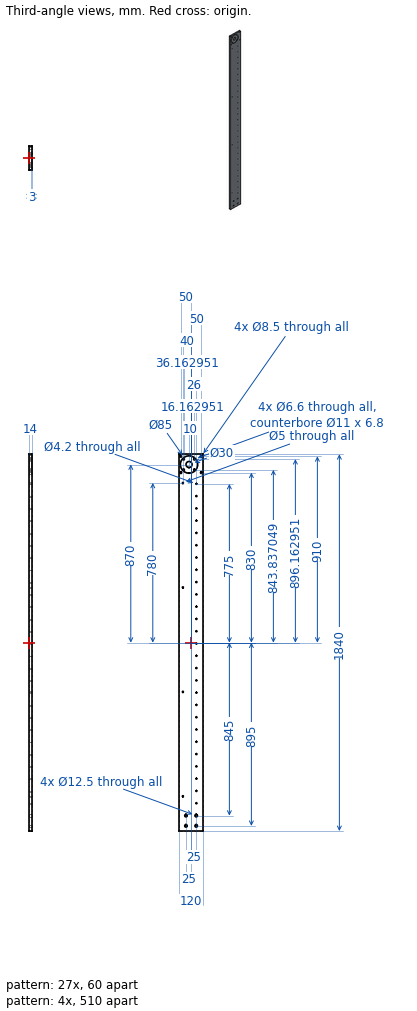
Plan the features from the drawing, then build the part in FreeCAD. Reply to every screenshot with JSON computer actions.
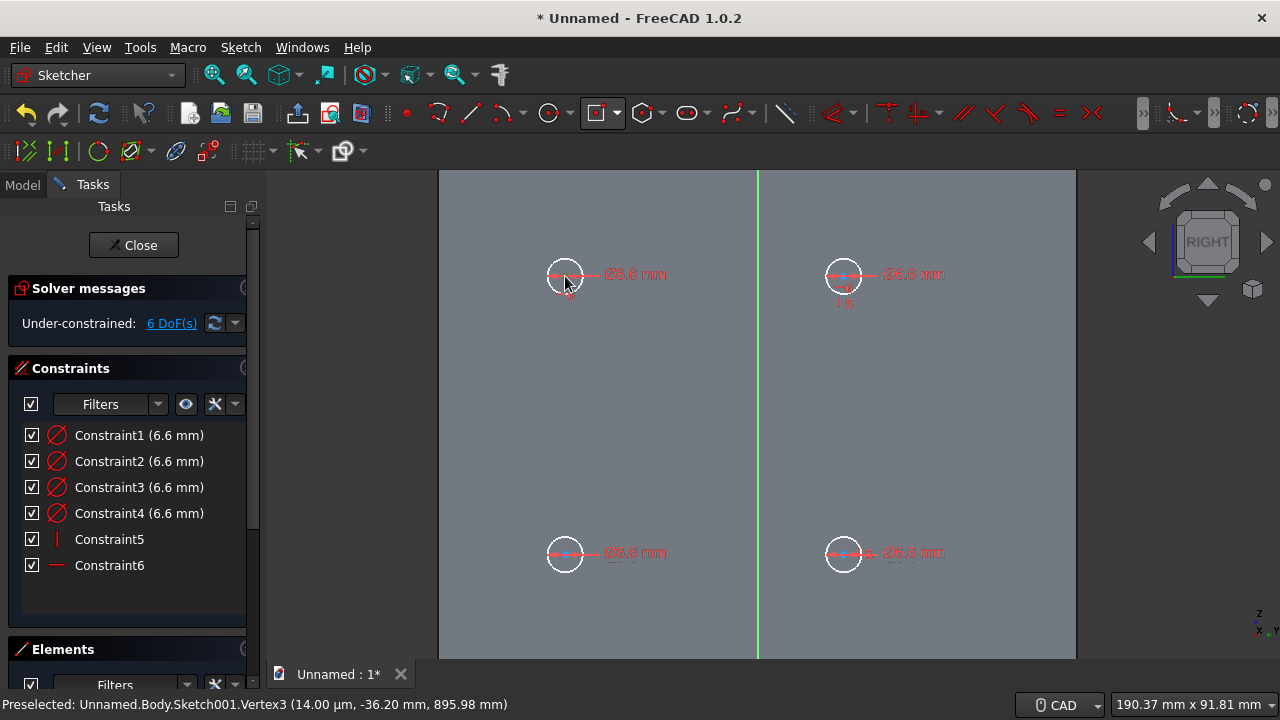
{"action": "left_click", "coordinate": [565, 555]}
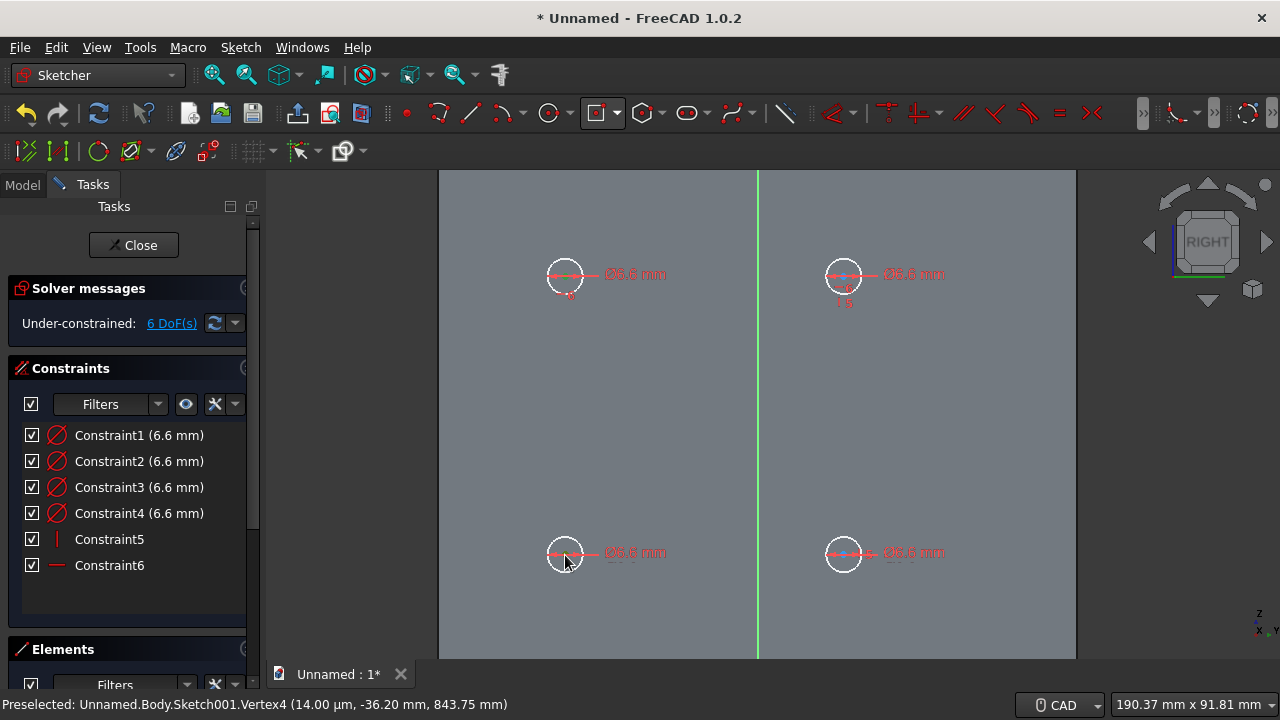
{"action": "key", "text": "v"}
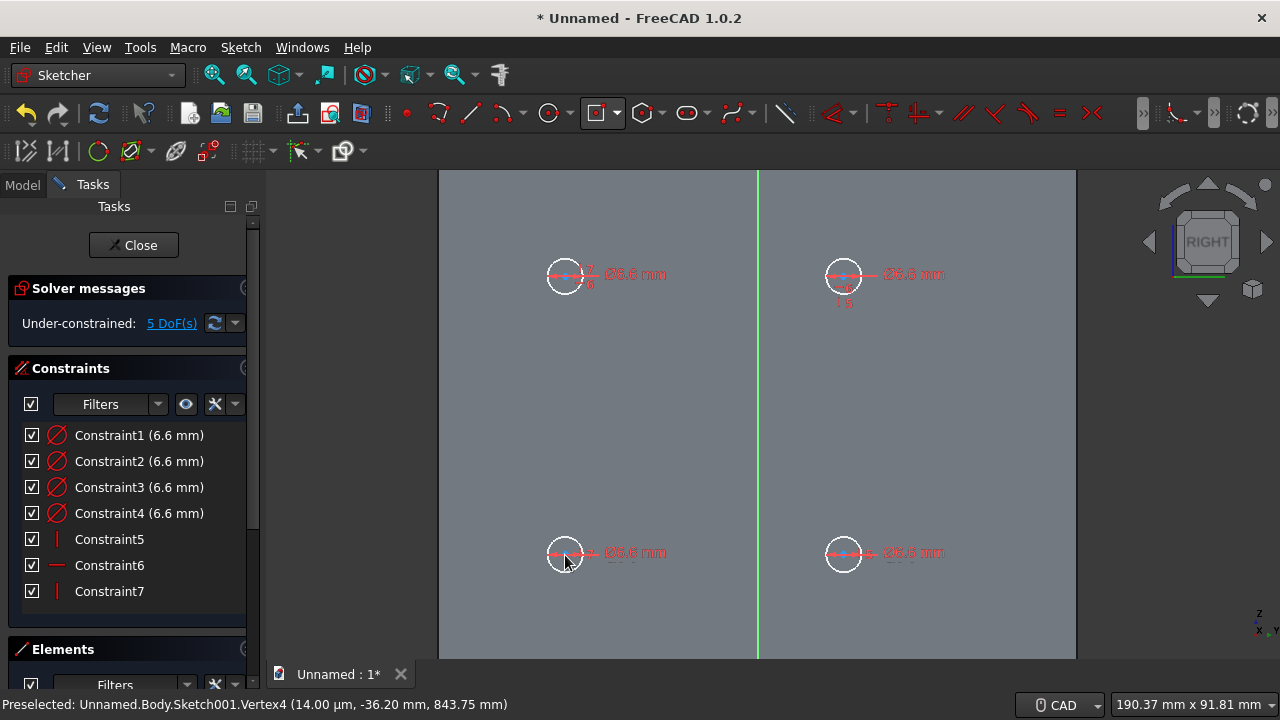
{"action": "left_click", "coordinate": [844, 555]}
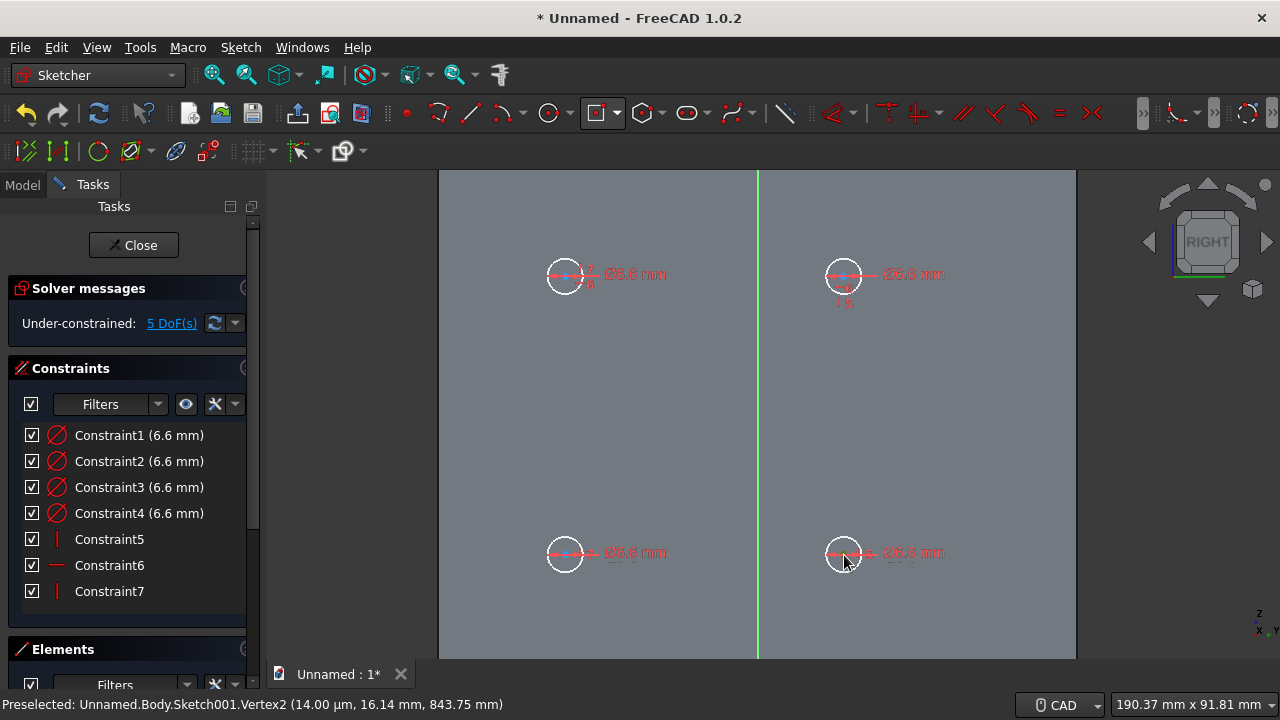
{"action": "left_click", "coordinate": [565, 555]}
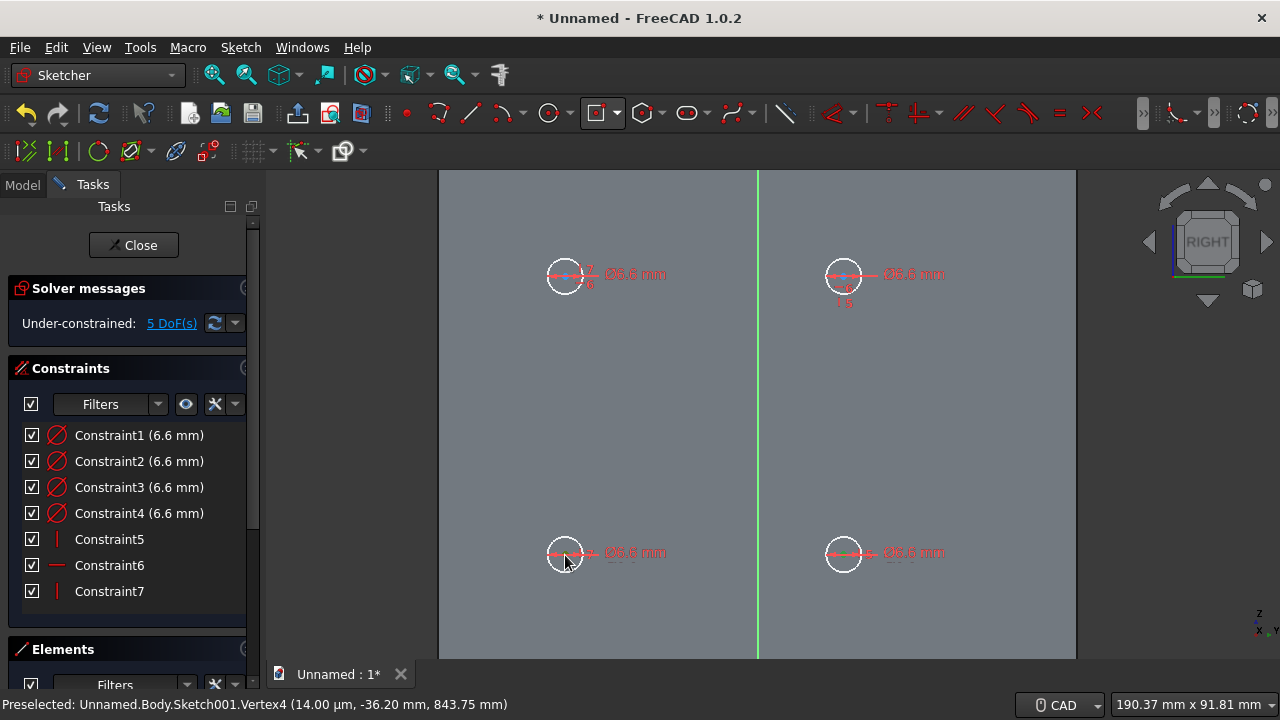
{"action": "key", "text": "h"}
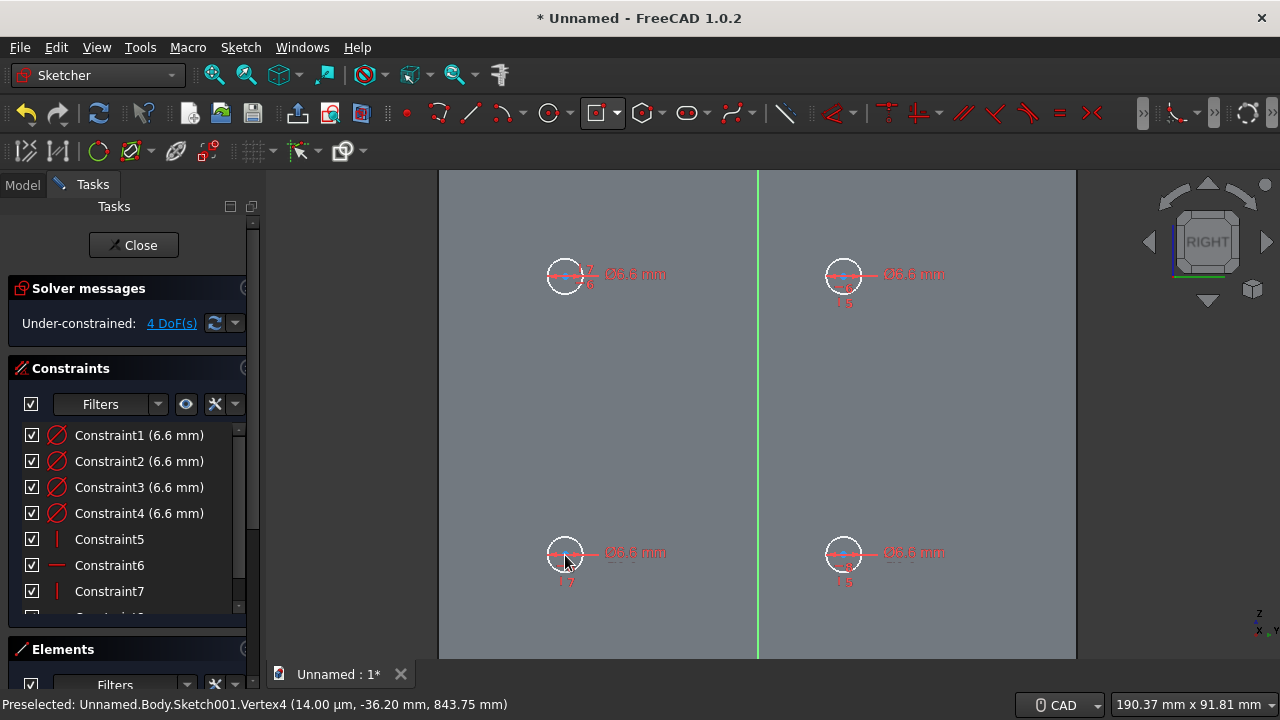
{"action": "left_click", "coordinate": [832, 114]}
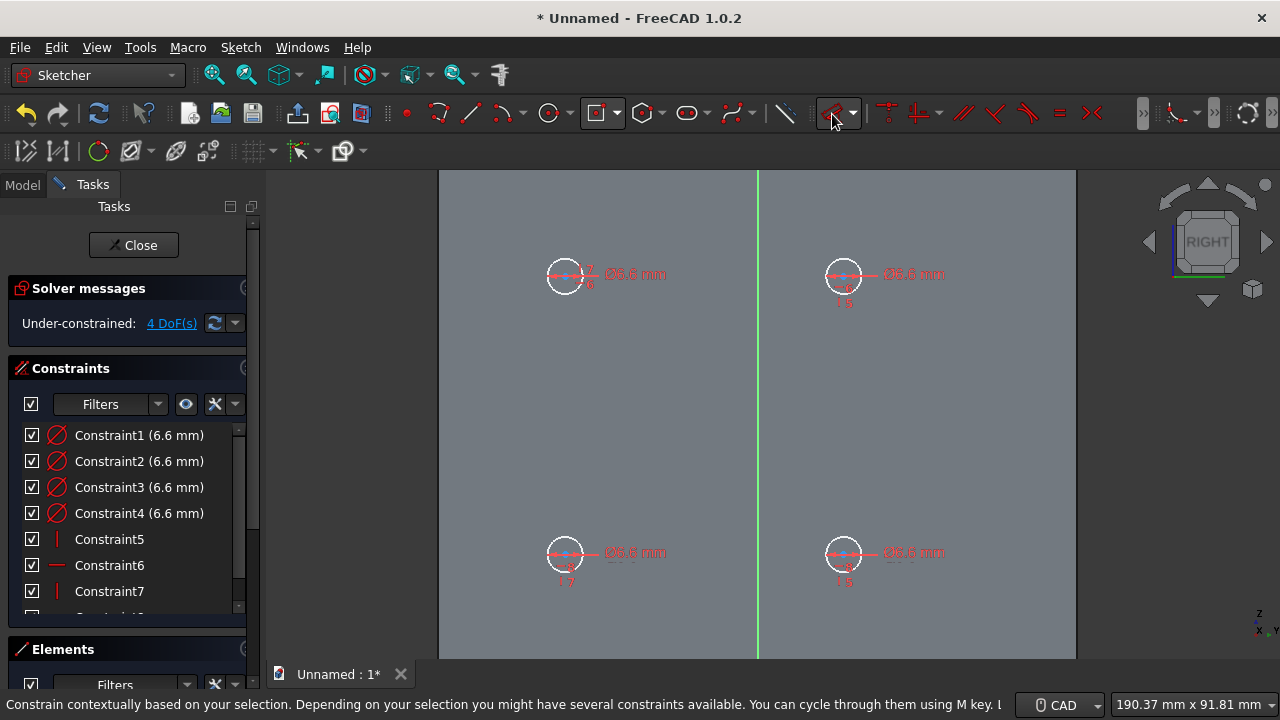
{"action": "left_click", "coordinate": [844, 276]}
{"action": "left_click", "coordinate": [801, 242]}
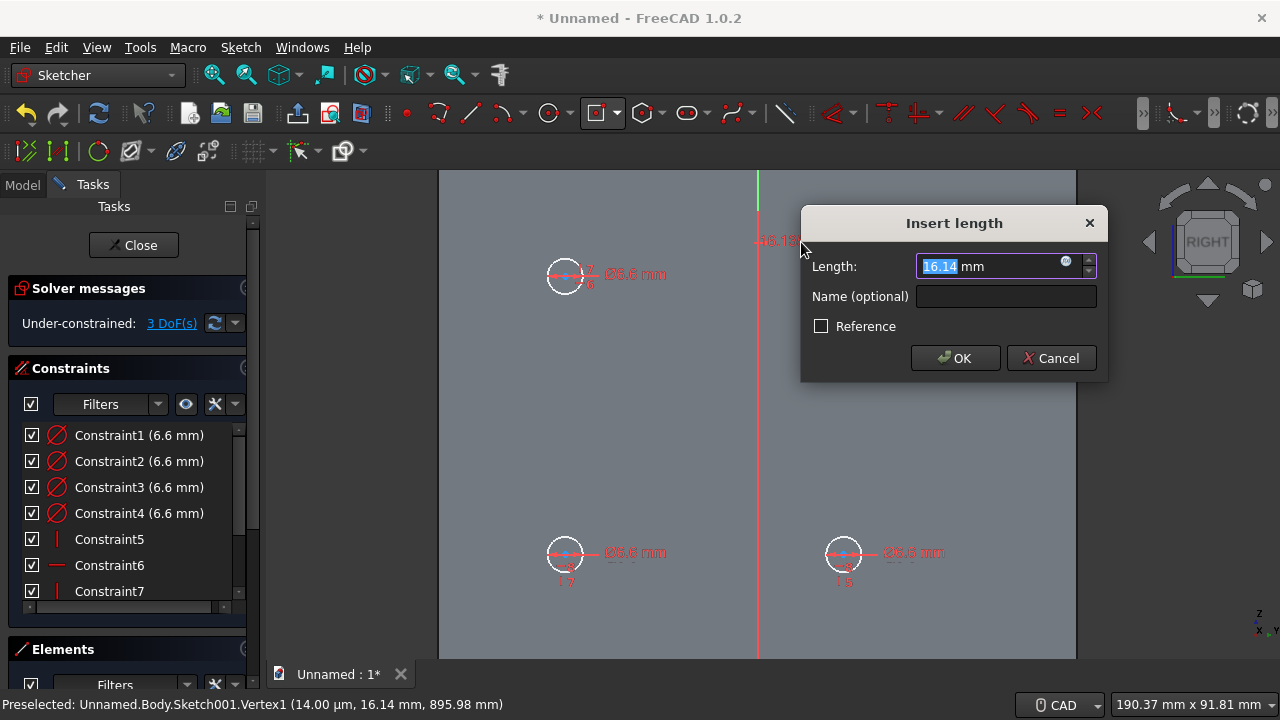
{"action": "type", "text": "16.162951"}
{"action": "key", "text": "Return"}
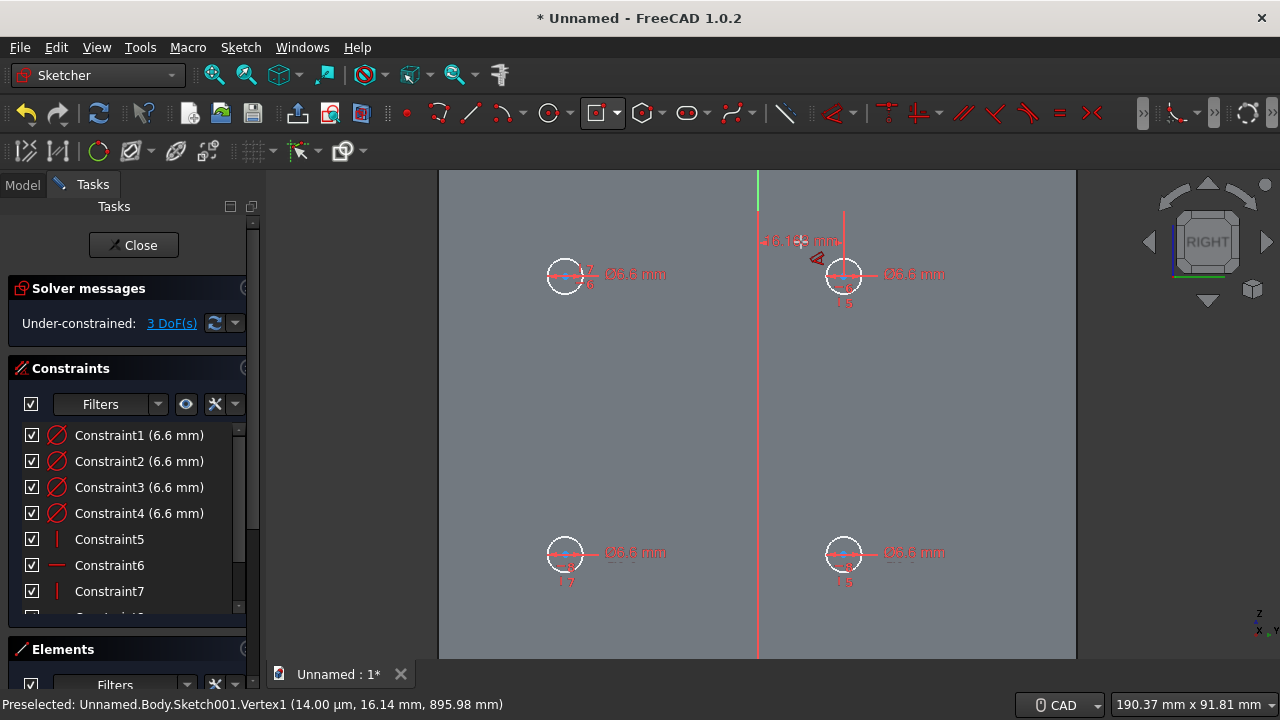
{"action": "left_click", "coordinate": [565, 276]}
{"action": "left_click", "coordinate": [661, 242]}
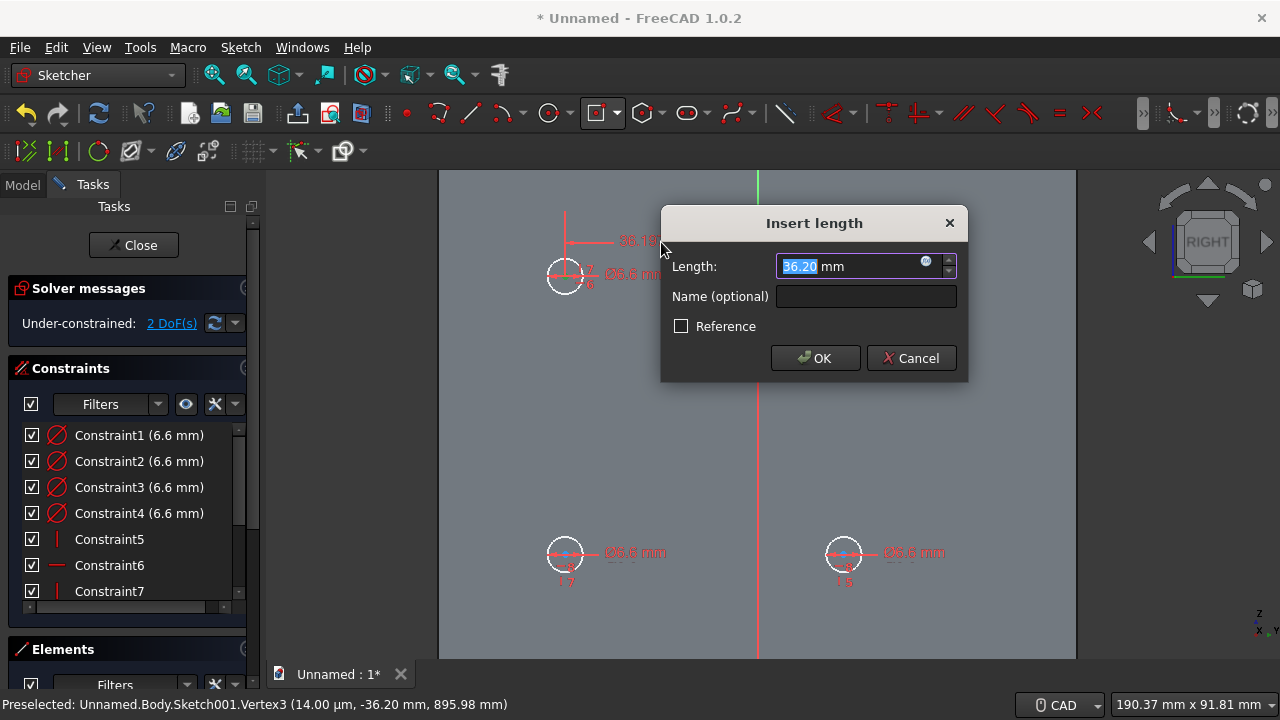
{"action": "type", "text": "36.162951"}
{"action": "key", "text": "Return"}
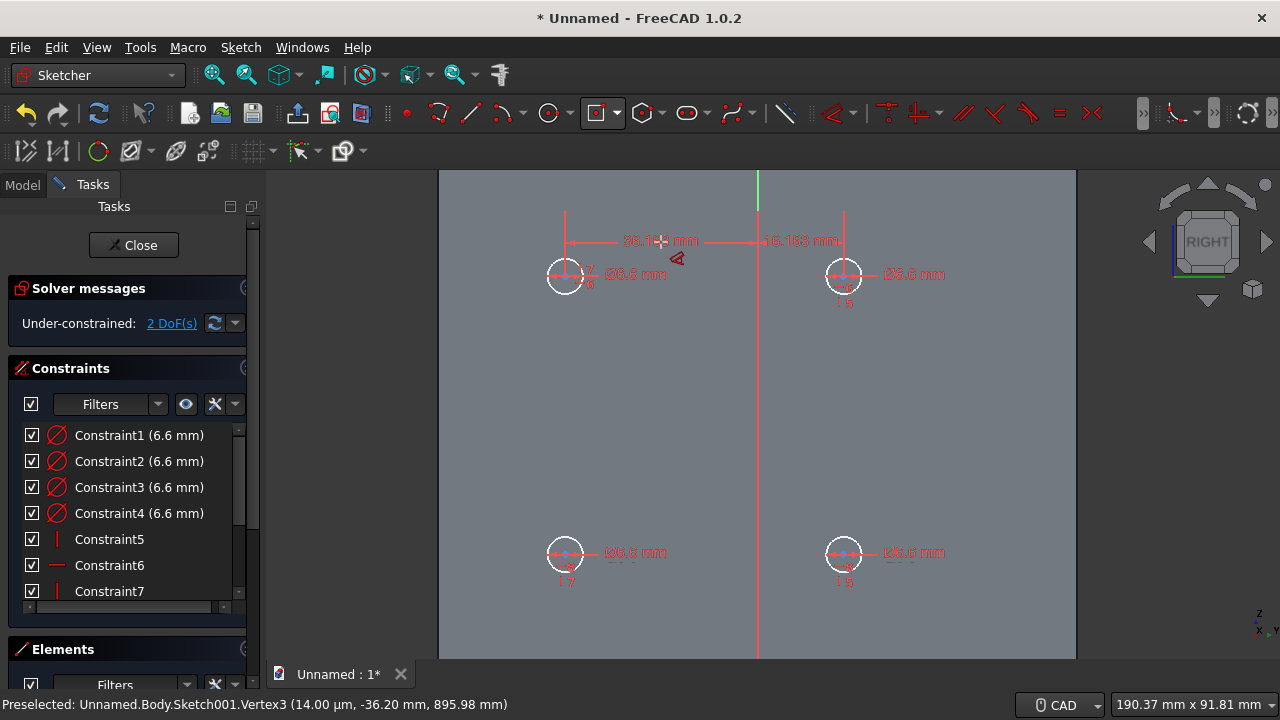
{"action": "left_click", "coordinate": [844, 276]}
{"action": "left_click", "coordinate": [878, 454]}